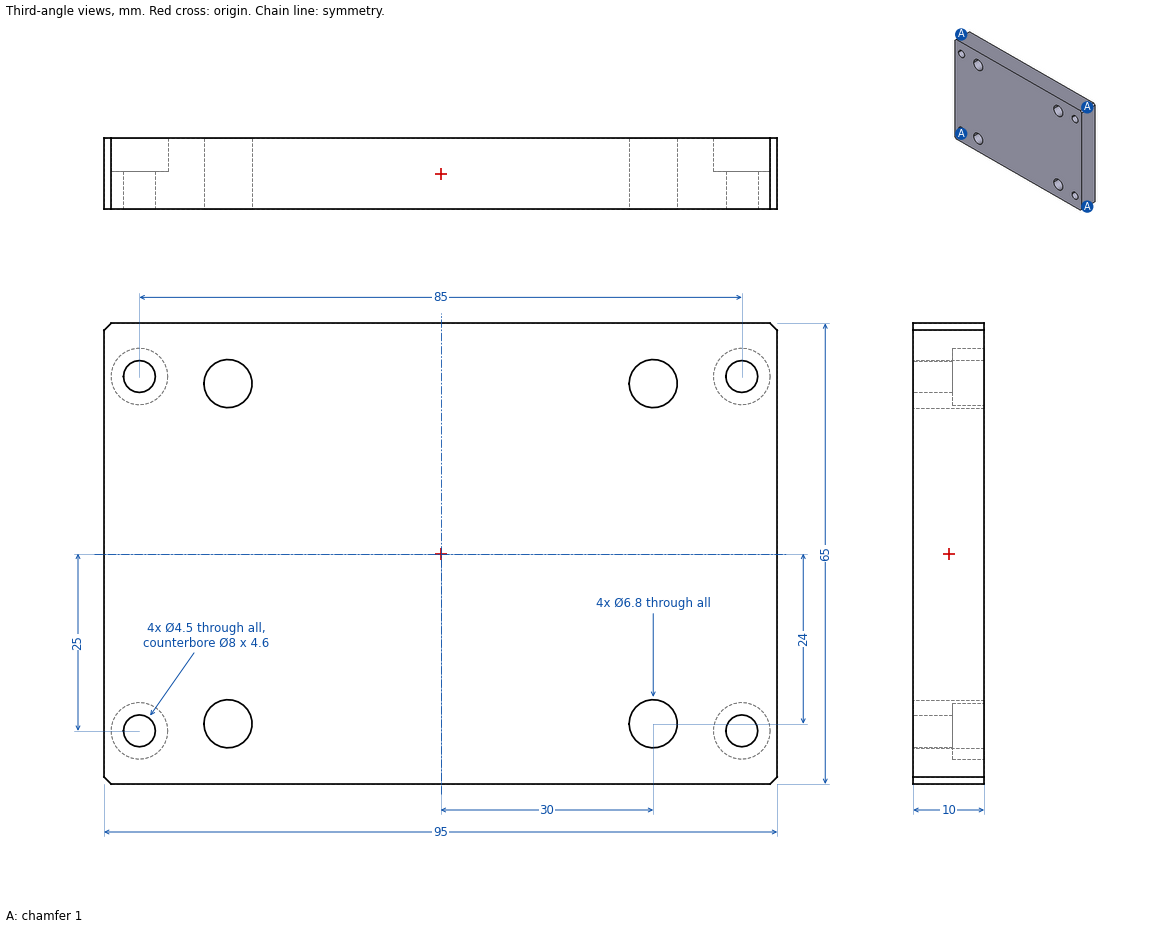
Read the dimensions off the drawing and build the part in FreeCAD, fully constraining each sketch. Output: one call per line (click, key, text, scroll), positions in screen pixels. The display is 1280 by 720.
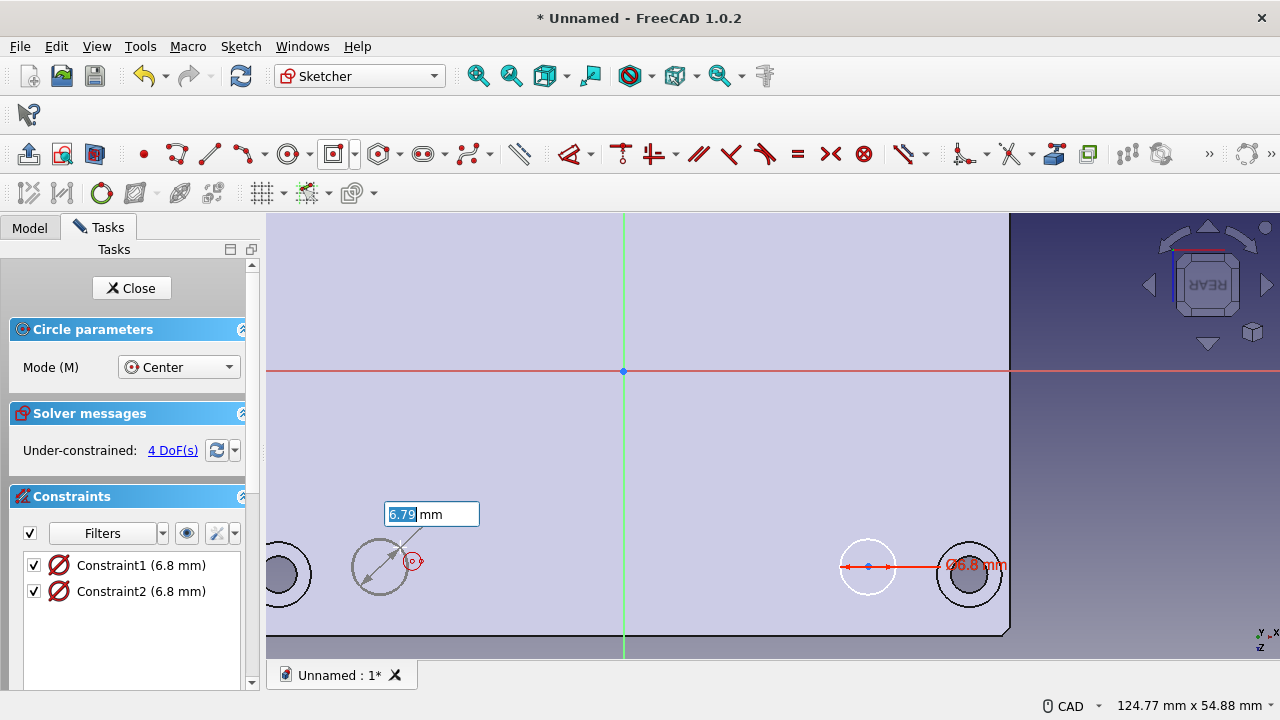
text(6.8)
key(Return)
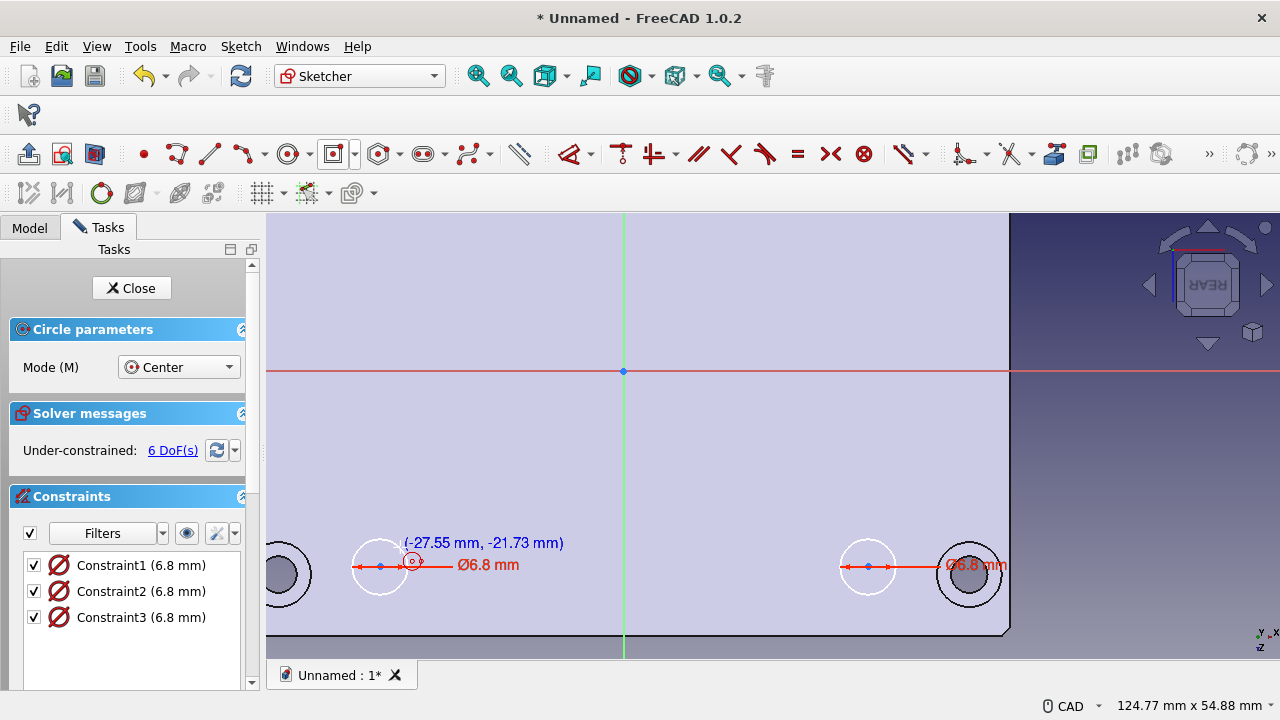
scroll(868, 567, down, 2)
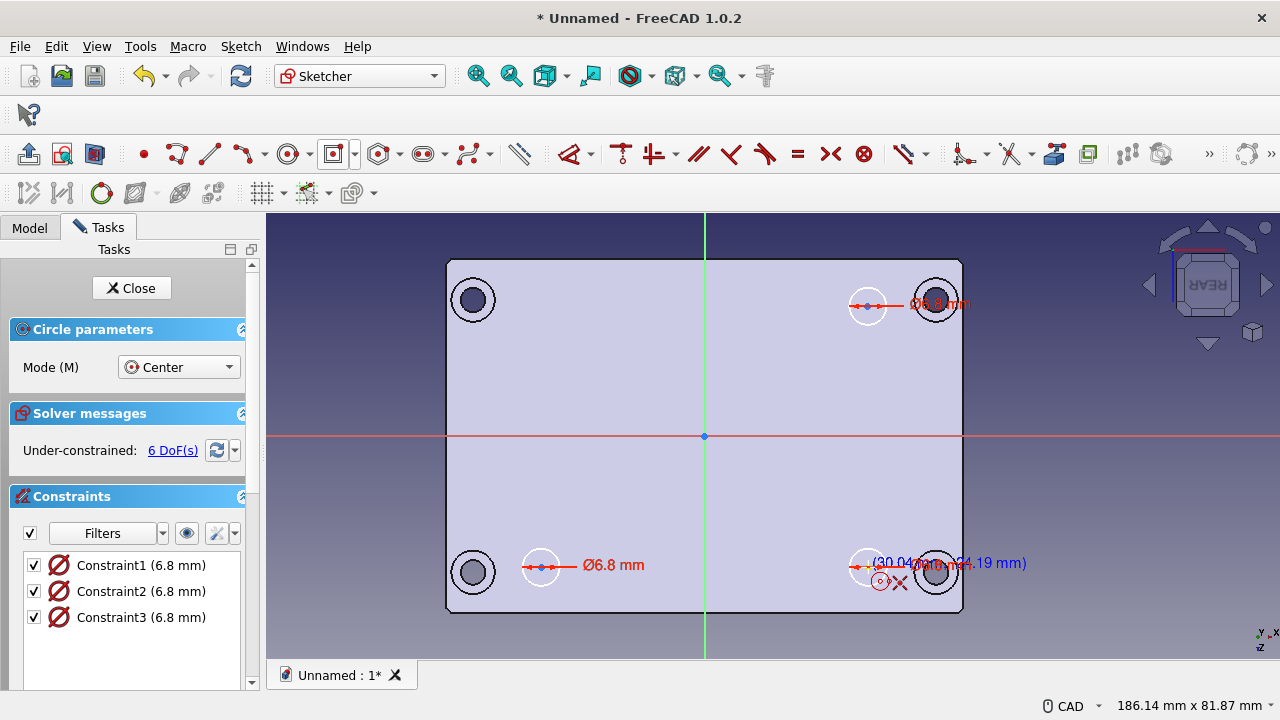
scroll(541, 305, up, 2)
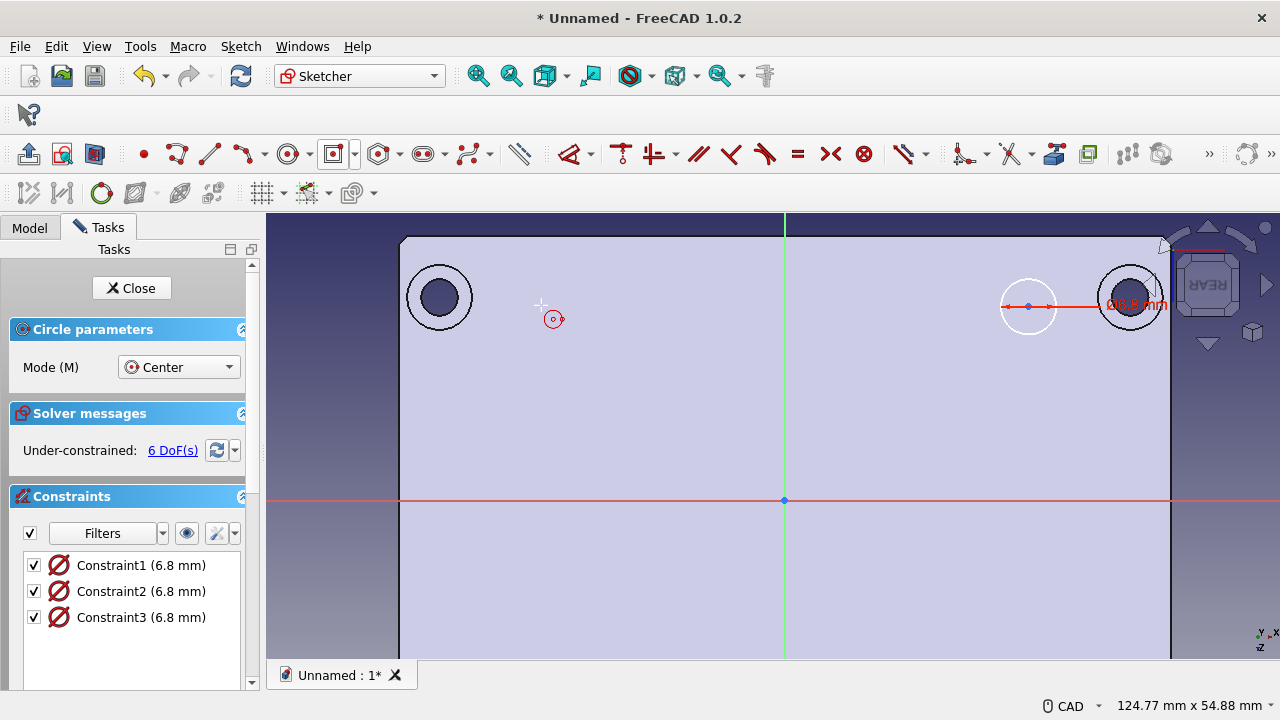
click(541, 306)
move(561, 286)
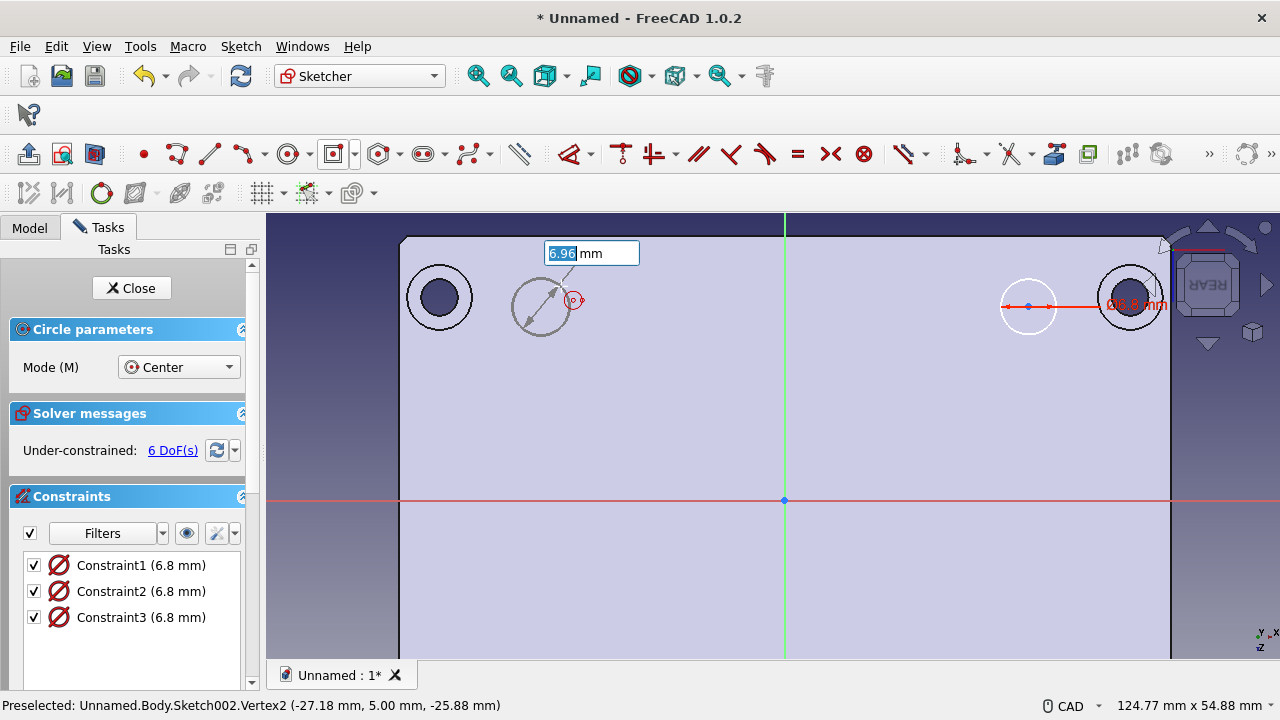
text(6.8)
key(Return)
key(Escape)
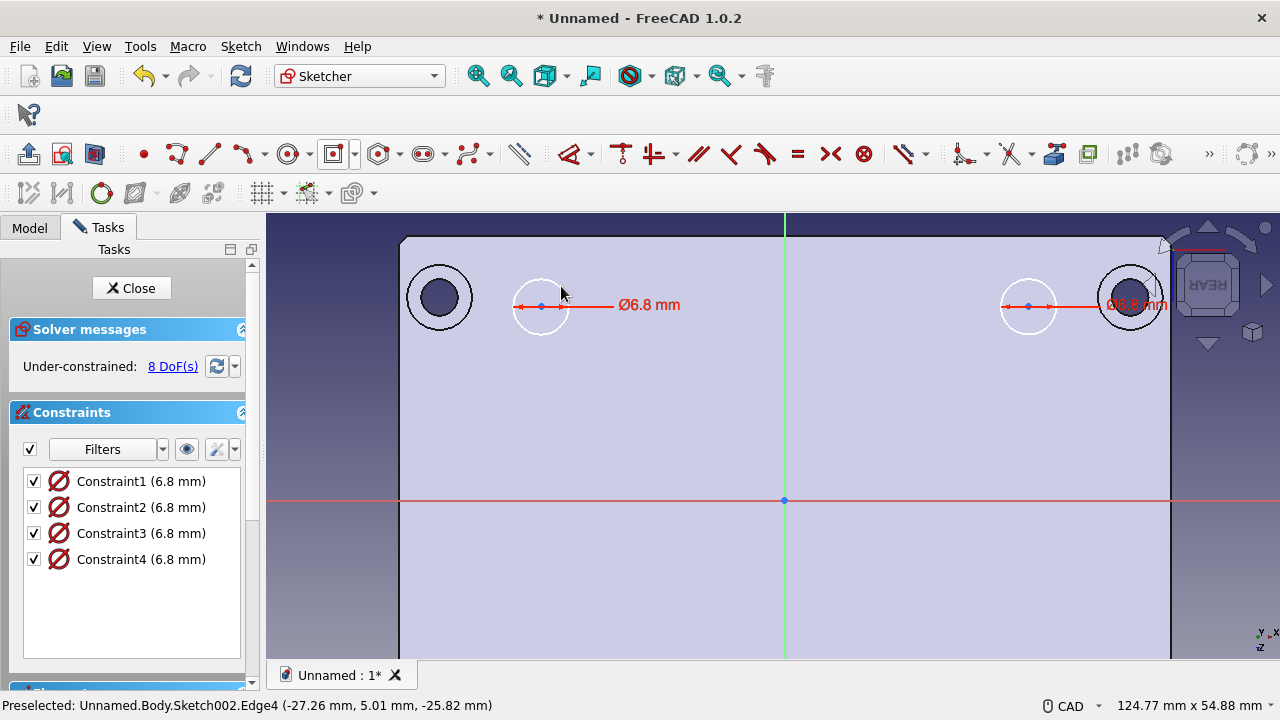
click(1029, 307)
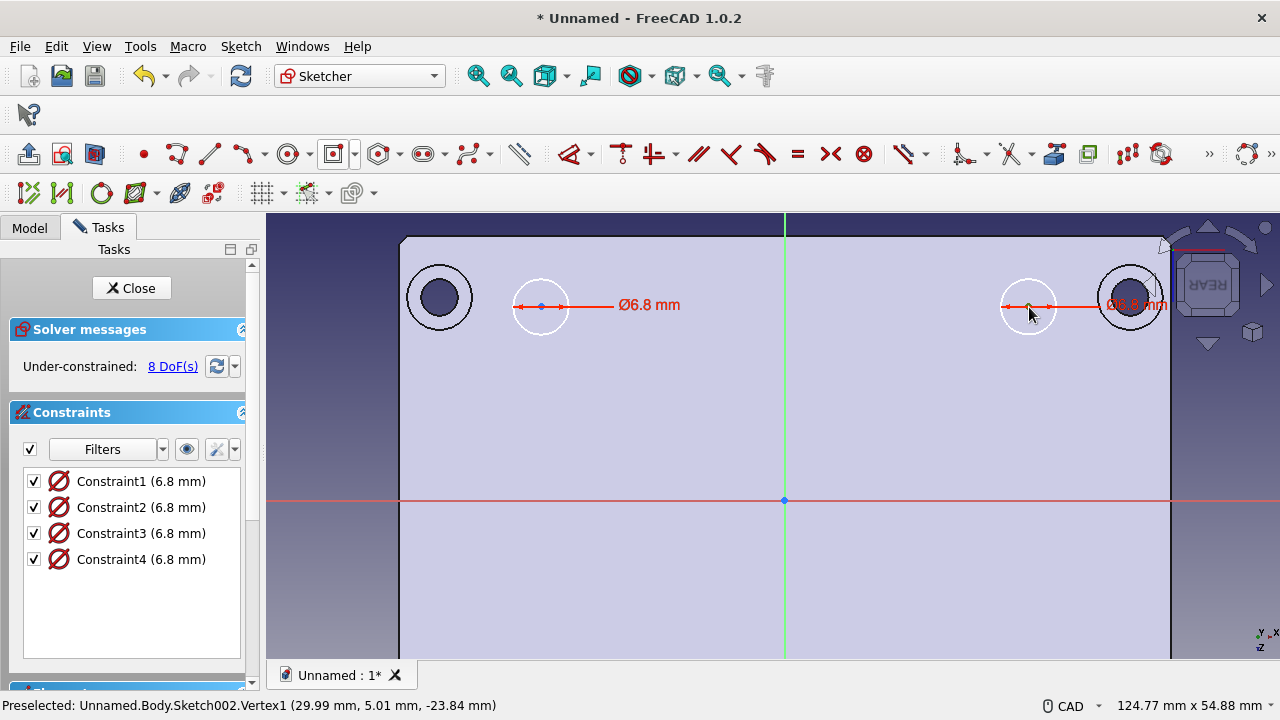
scroll(541, 305, down, 2)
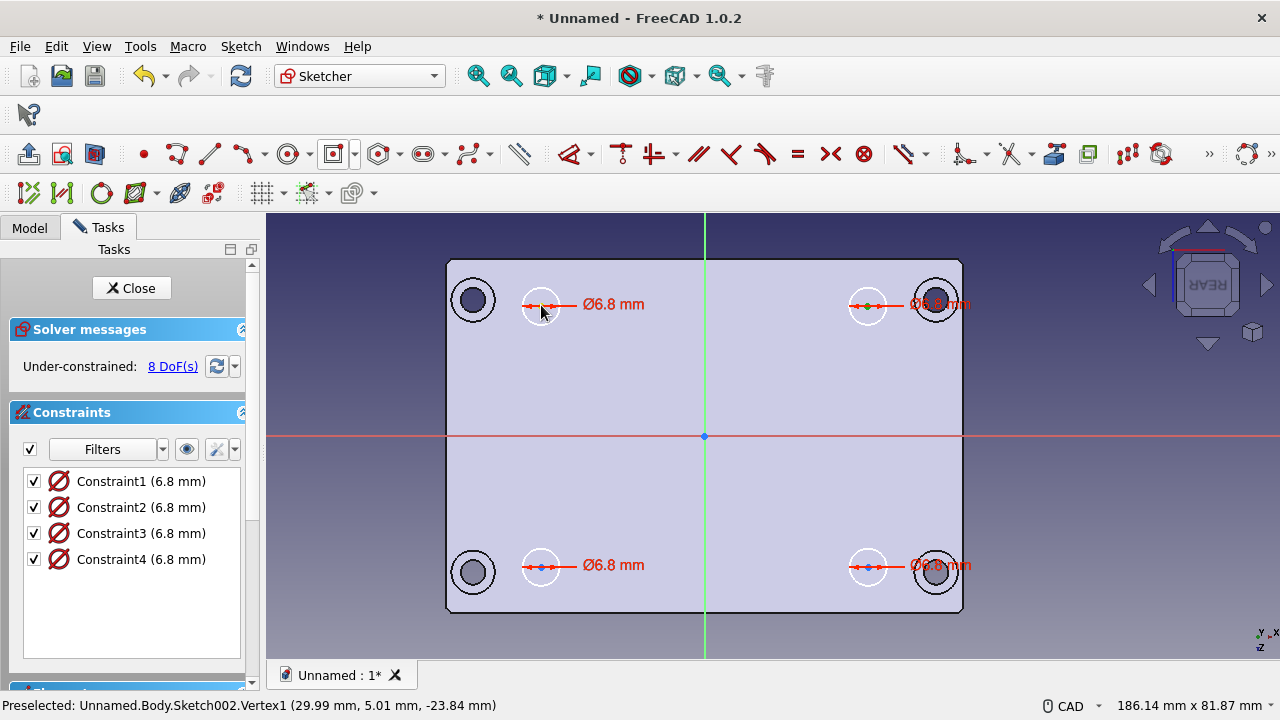
click(868, 567)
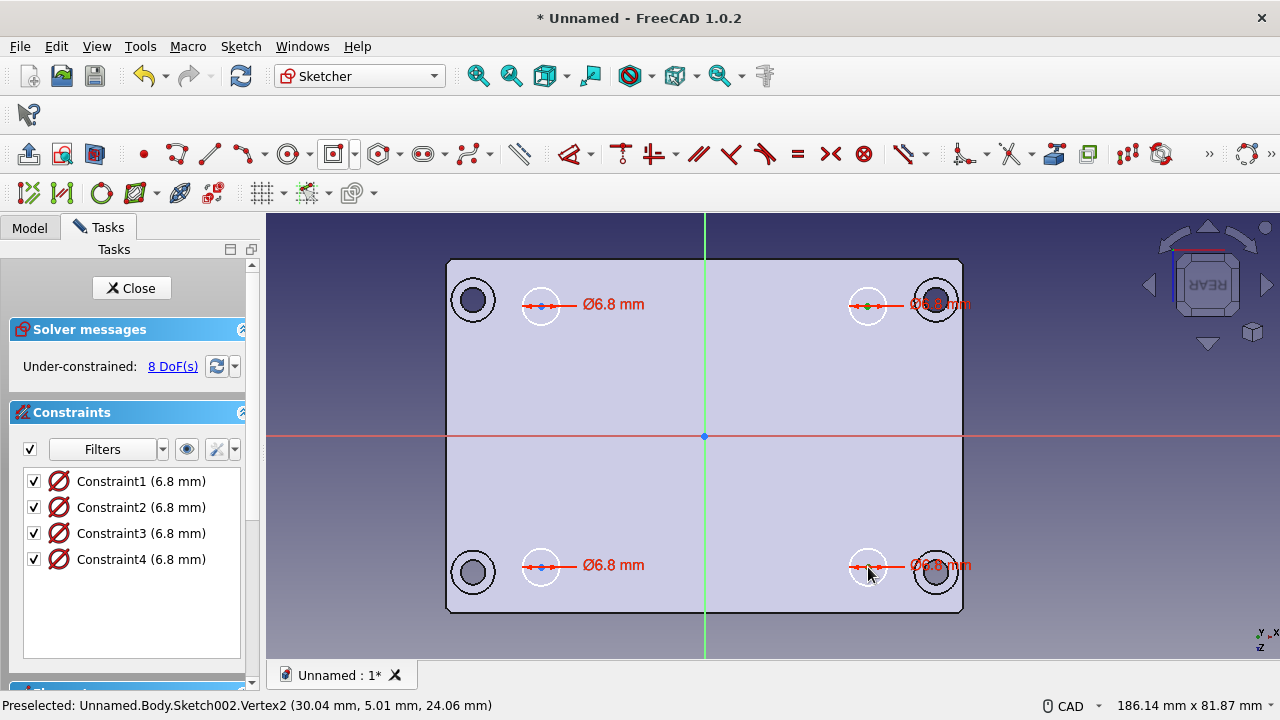
click(353, 436)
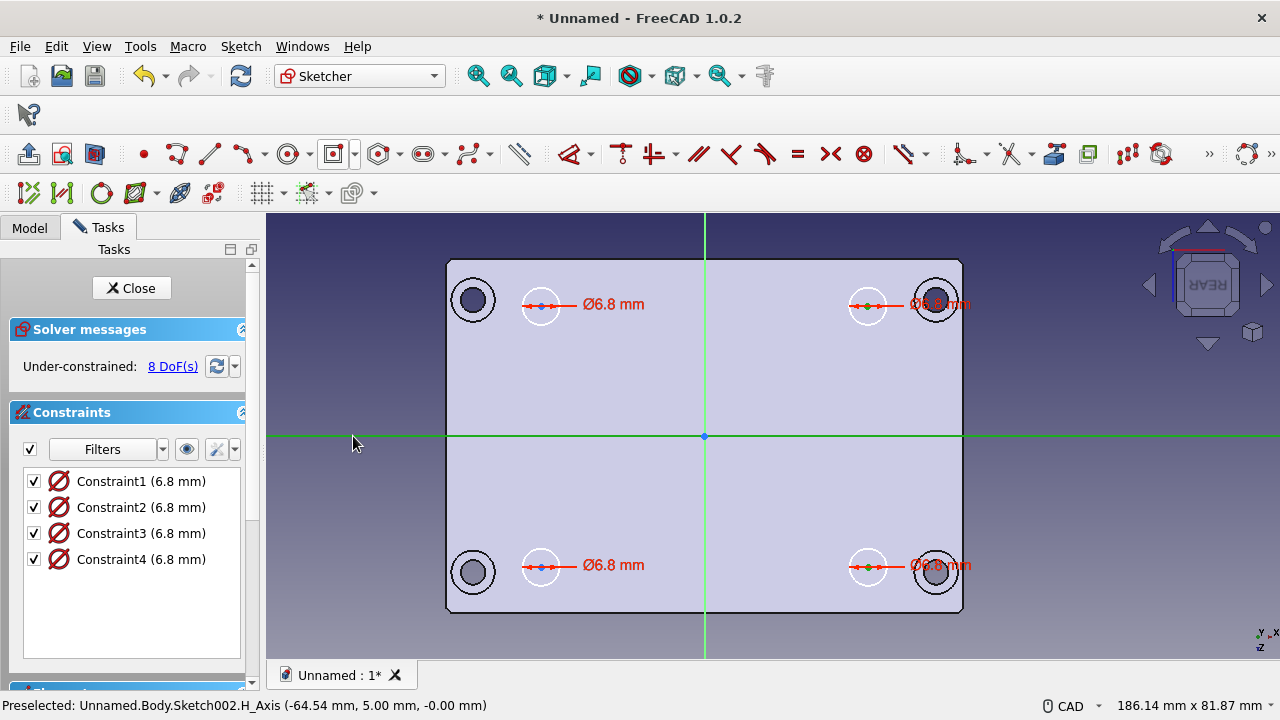
click(831, 154)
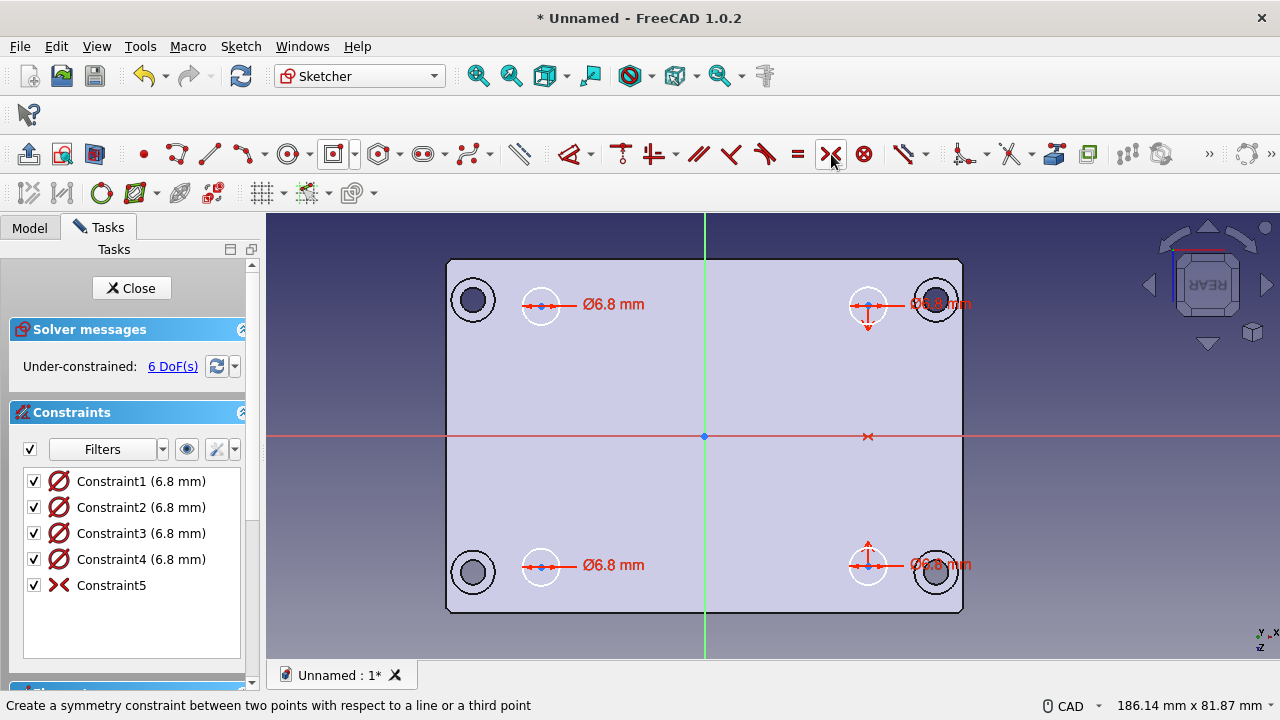
click(868, 566)